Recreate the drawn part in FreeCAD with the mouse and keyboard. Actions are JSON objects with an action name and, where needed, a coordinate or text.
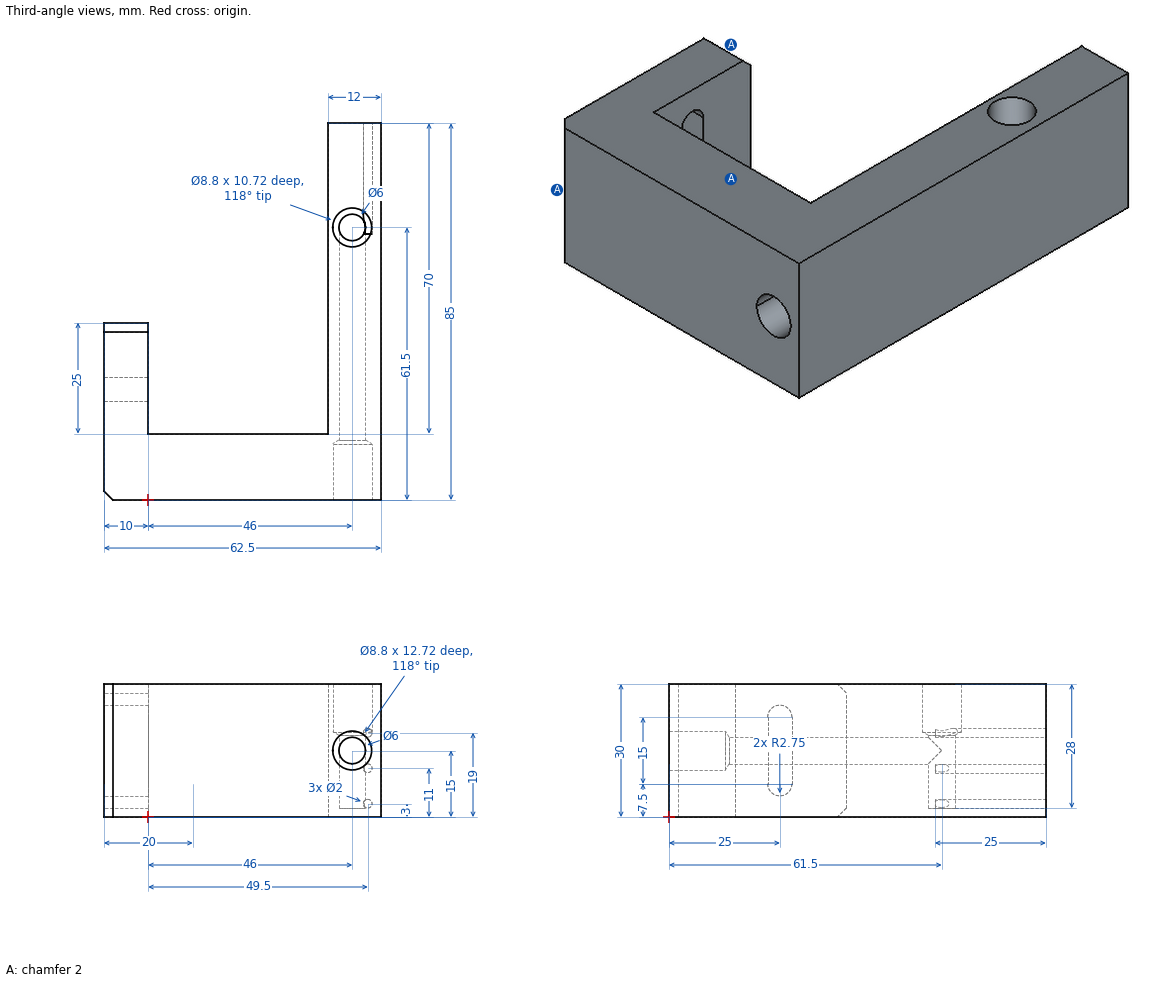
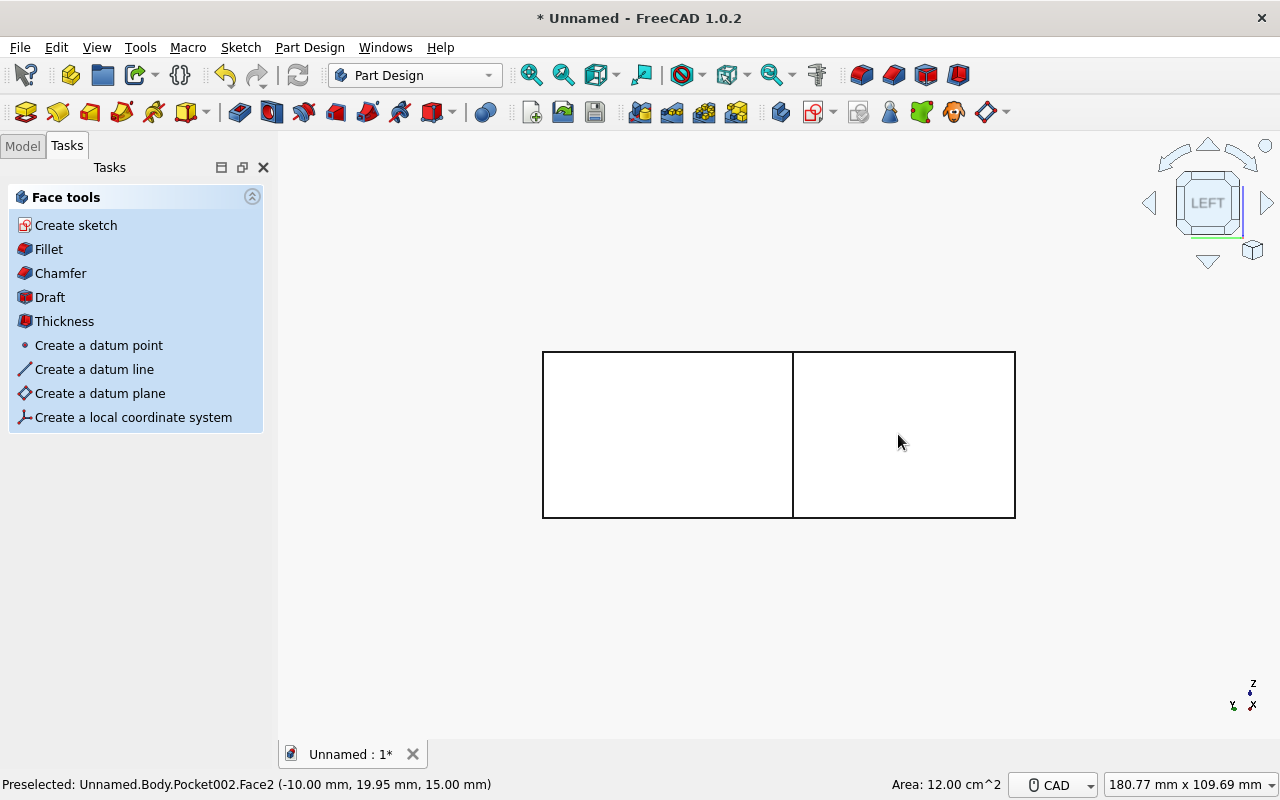
{"action": "left_click", "coordinate": [814, 112]}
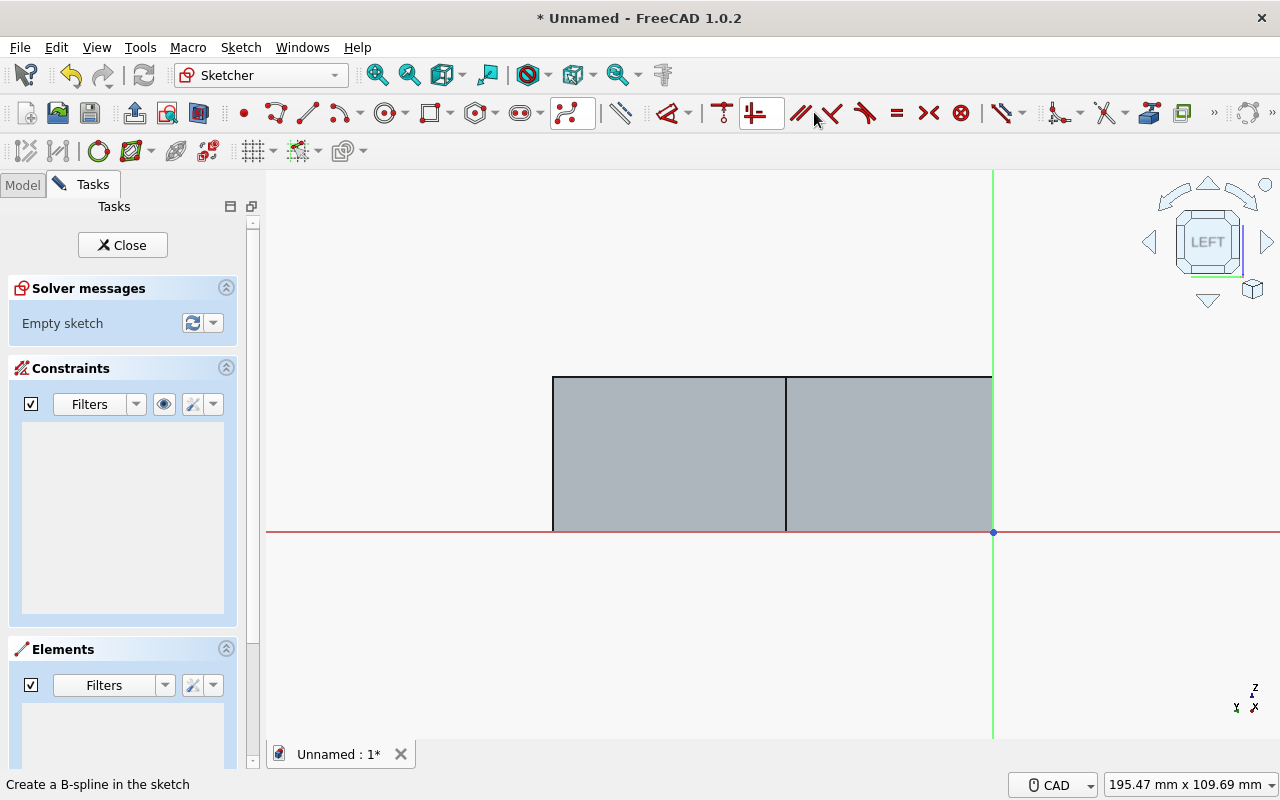
{"action": "scroll", "coordinate": [1048, 474], "scroll_direction": "up", "scroll_amount": 5}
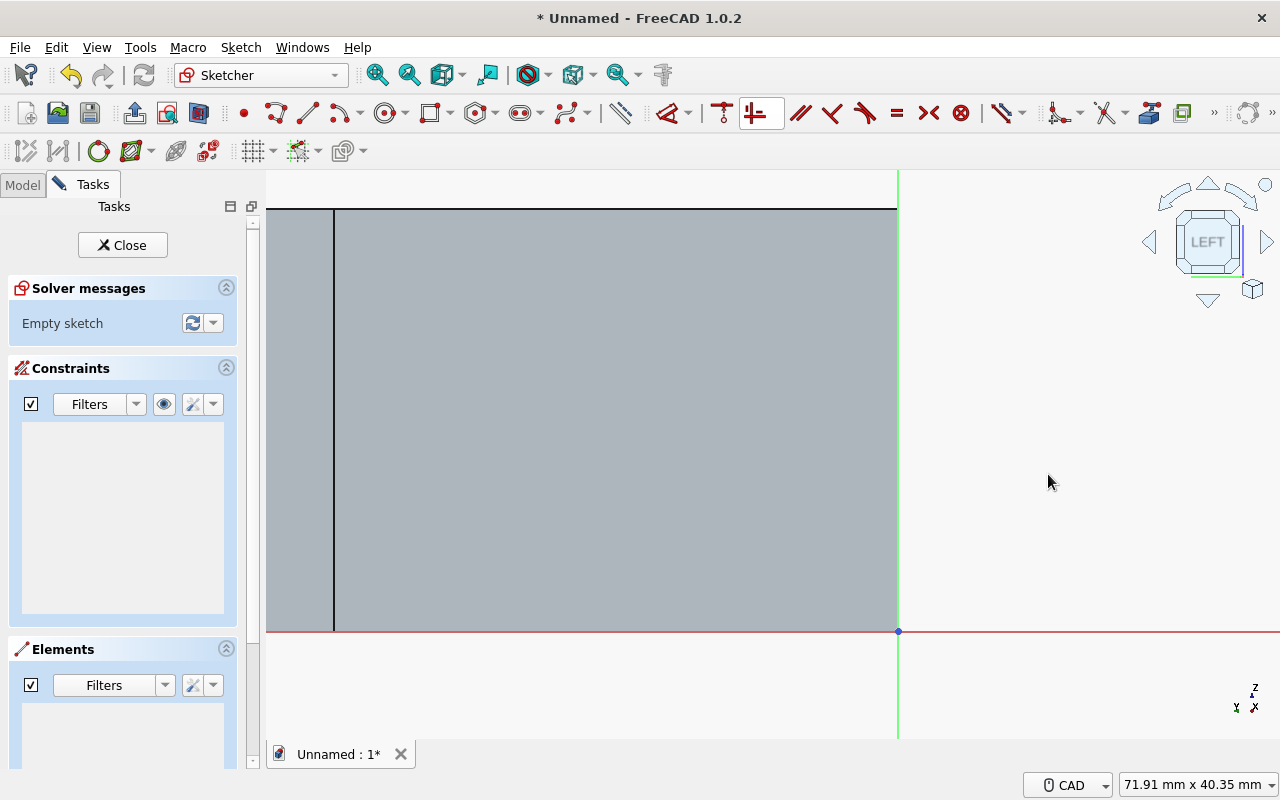
{"action": "left_click", "coordinate": [520, 114]}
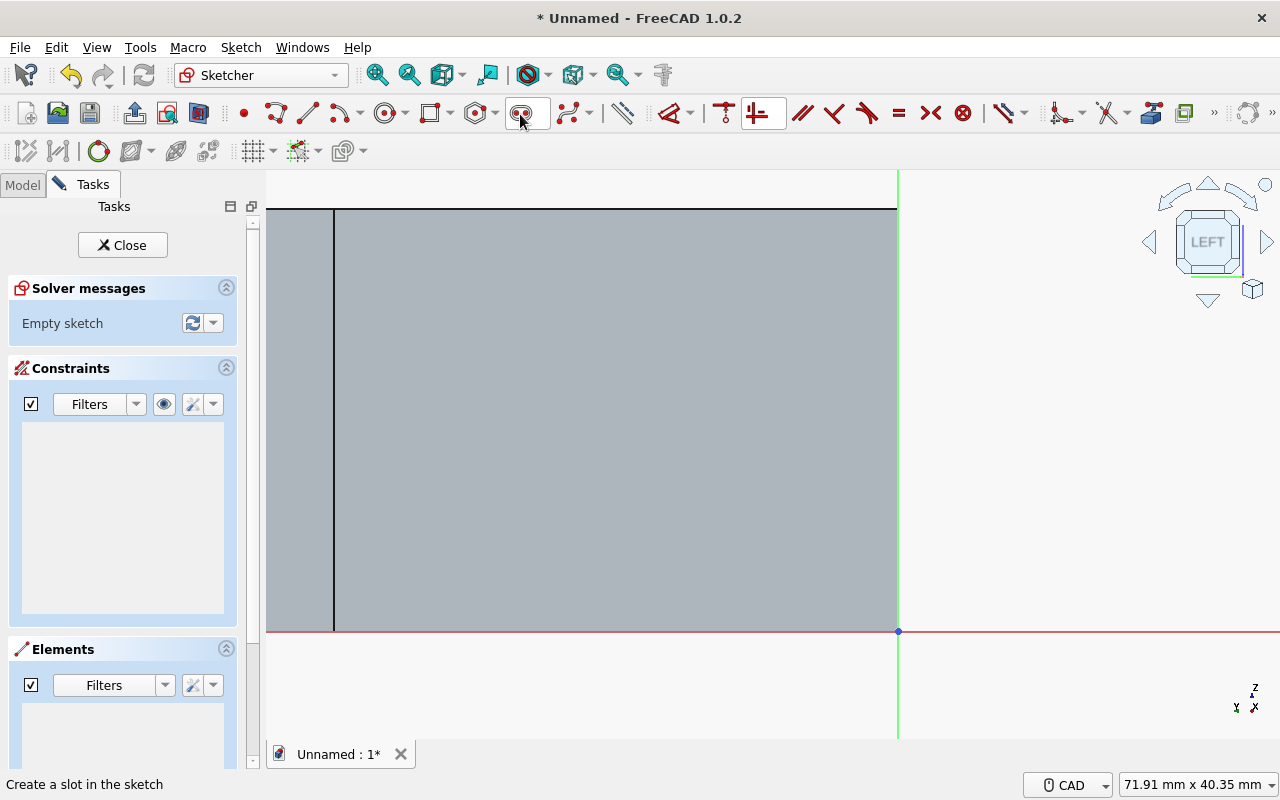
{"action": "left_click", "coordinate": [546, 526]}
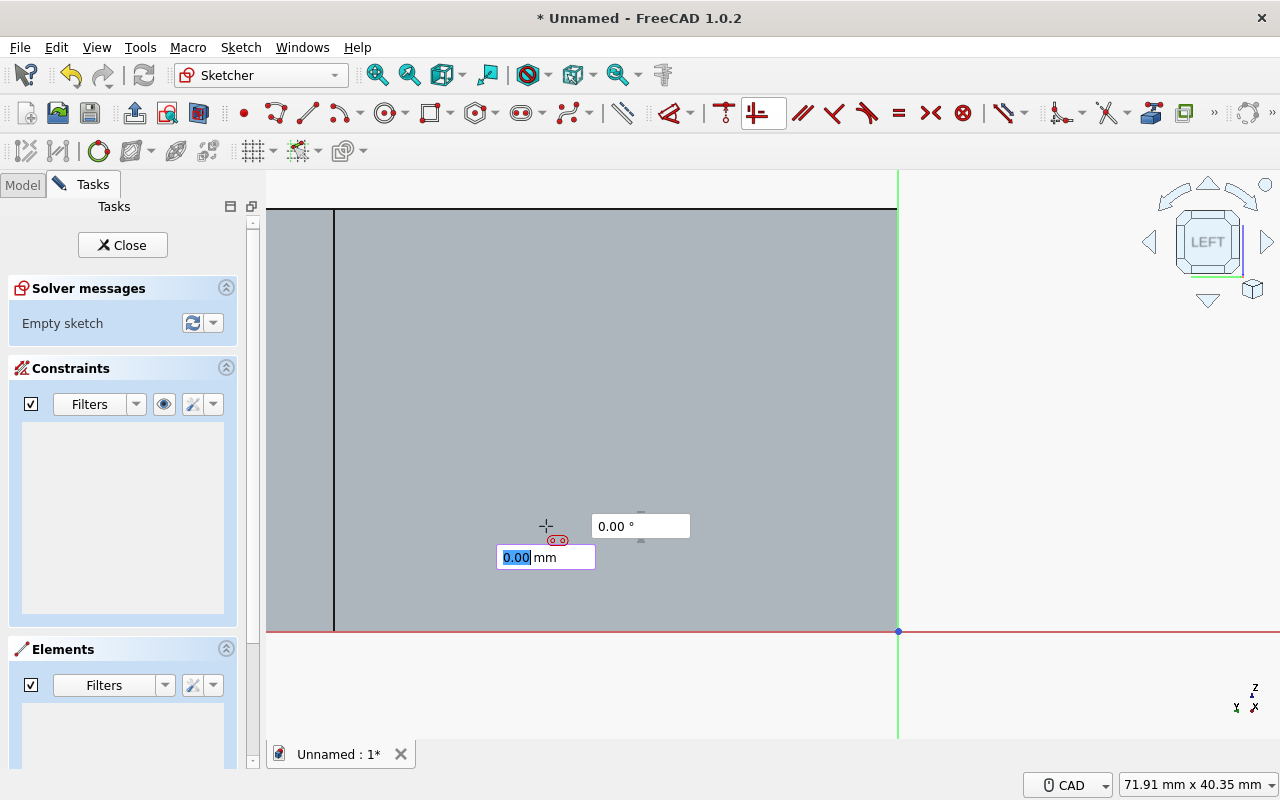
{"action": "left_click", "coordinate": [546, 314]}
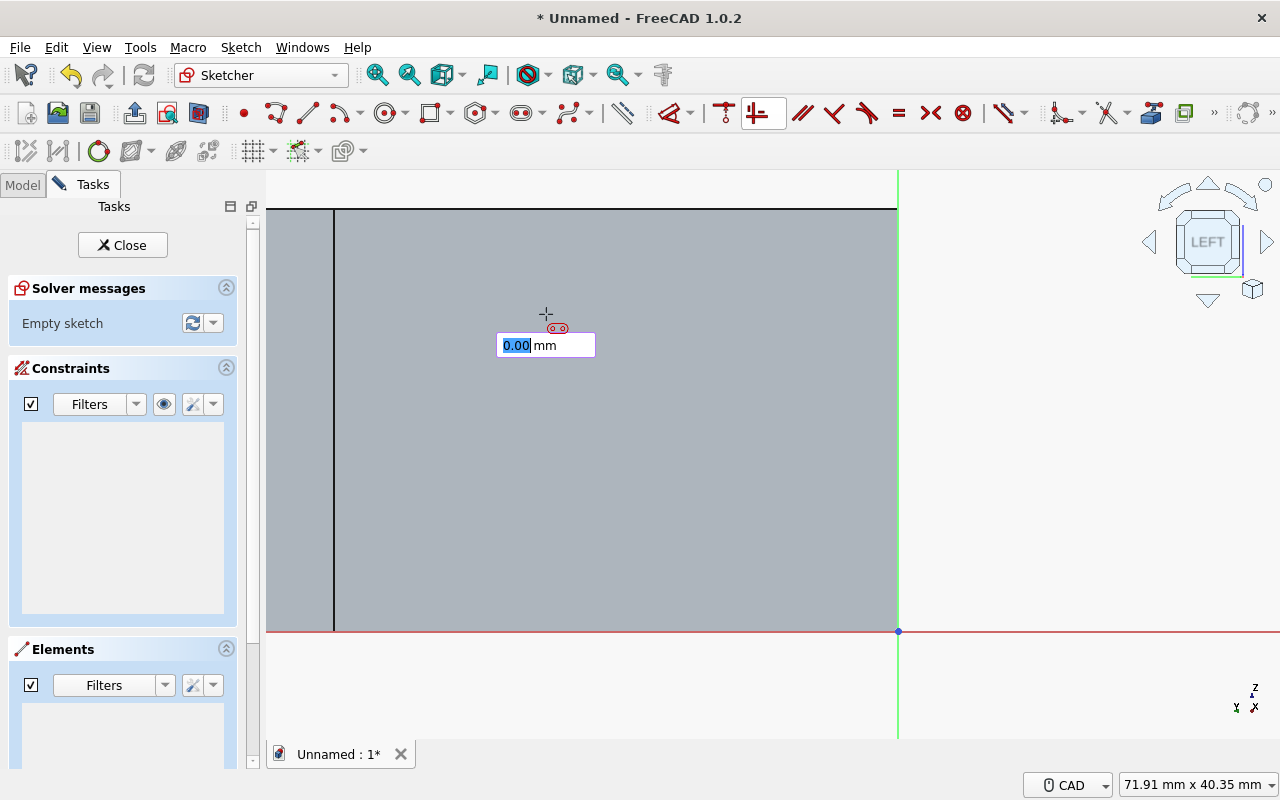
{"action": "left_click", "coordinate": [507, 420]}
{"action": "key", "text": "Escape"}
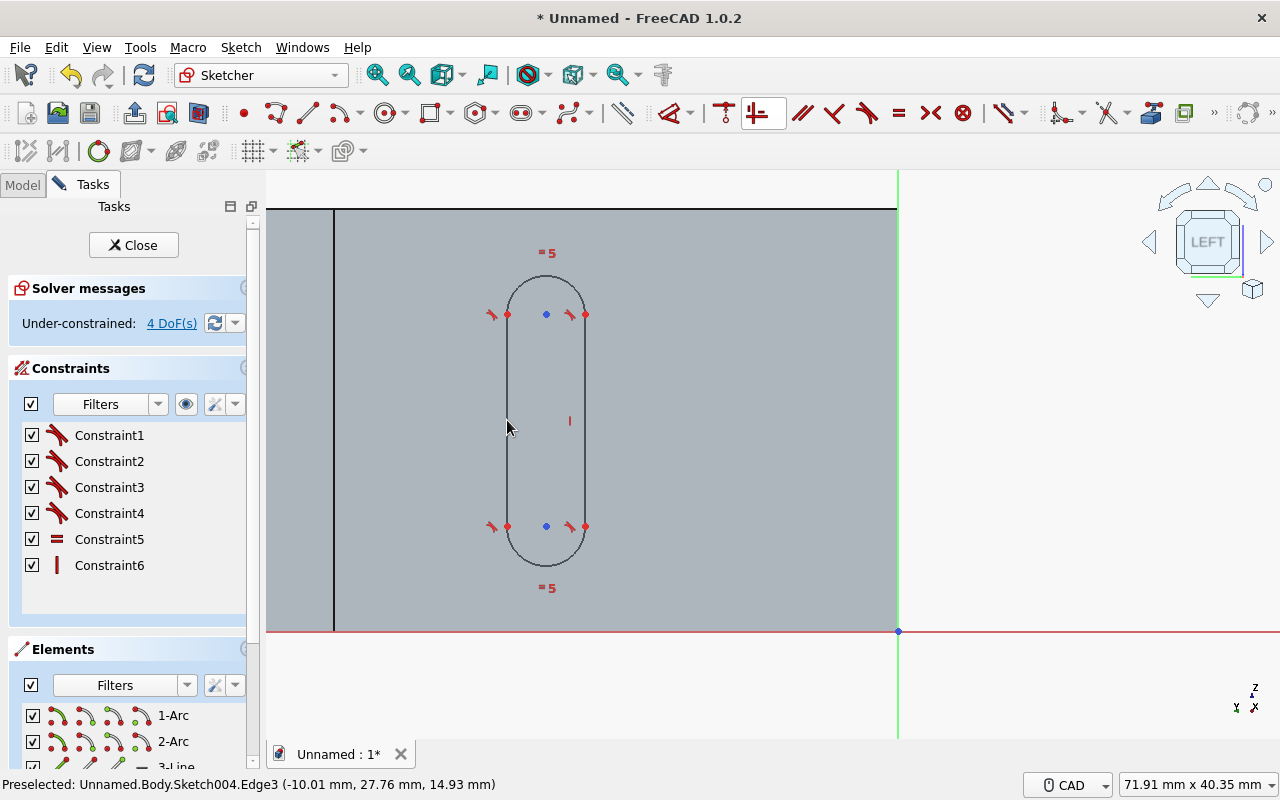
{"action": "left_click", "coordinate": [670, 114]}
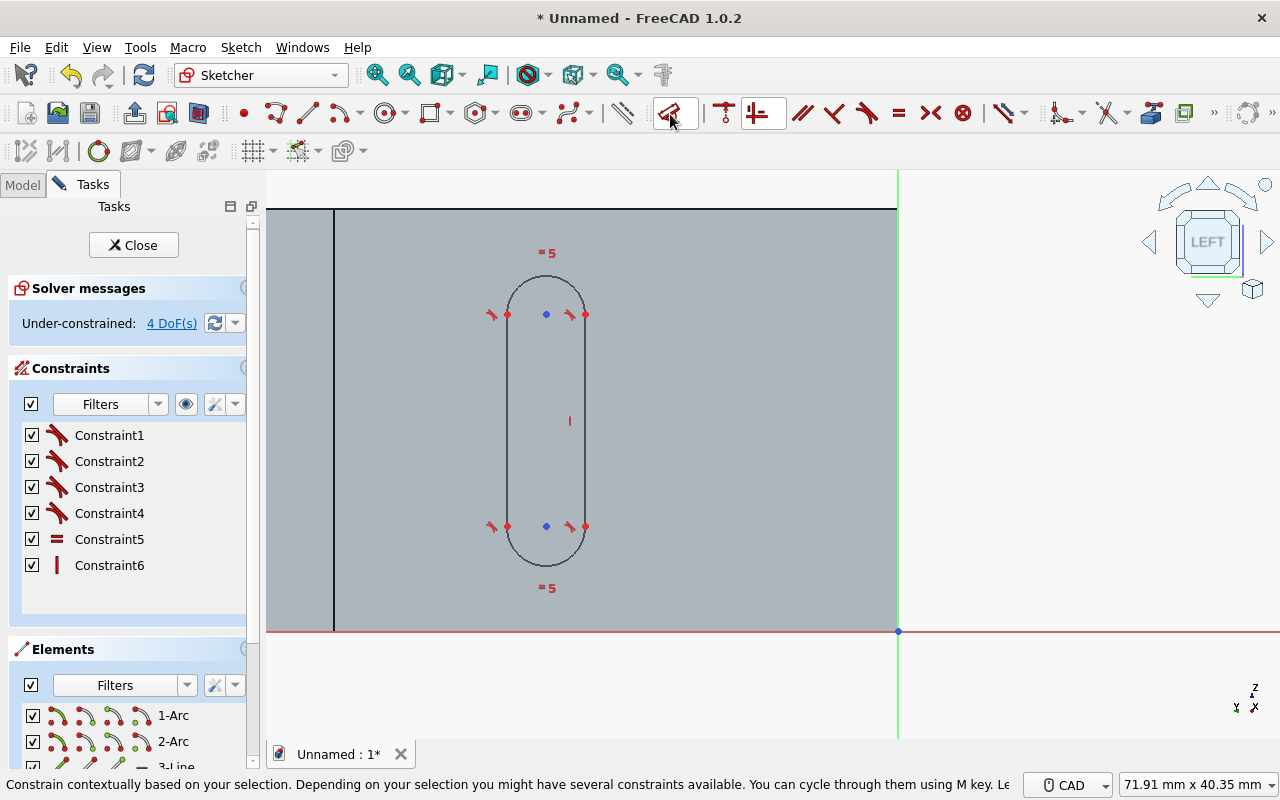
{"action": "left_click", "coordinate": [523, 559]}
{"action": "left_click", "coordinate": [504, 585]}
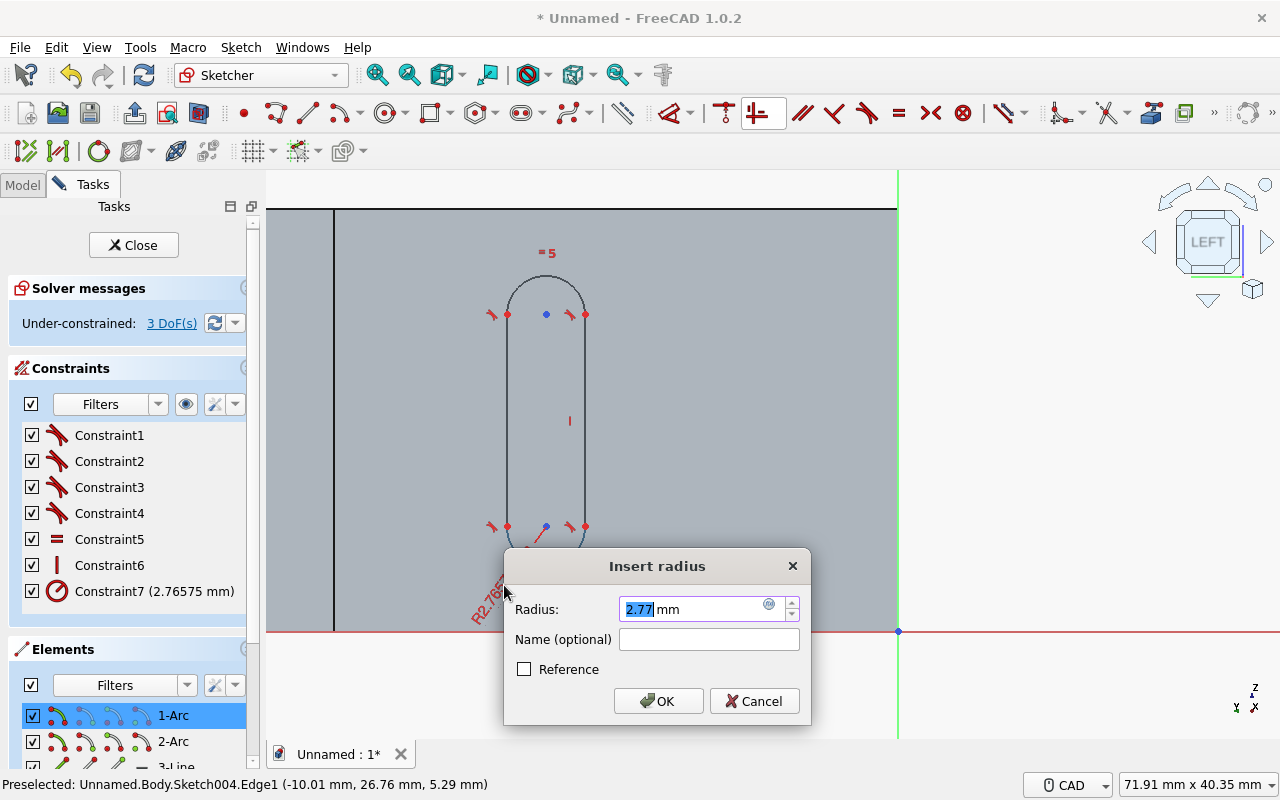
{"action": "type", "text": "2.75"}
{"action": "key", "text": "Return"}